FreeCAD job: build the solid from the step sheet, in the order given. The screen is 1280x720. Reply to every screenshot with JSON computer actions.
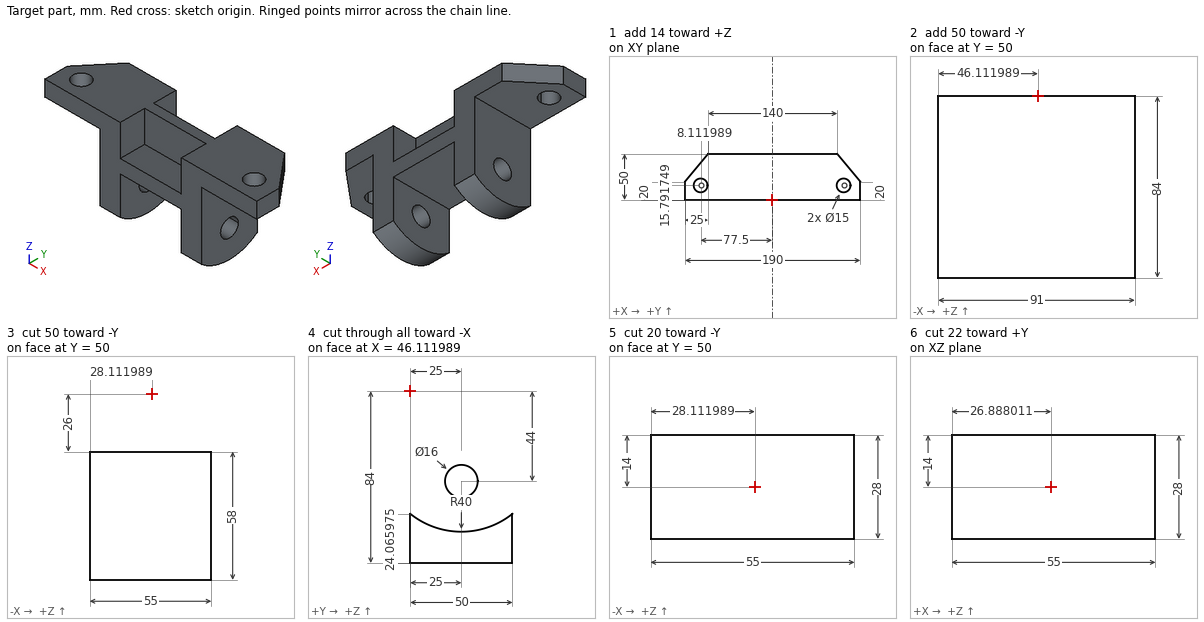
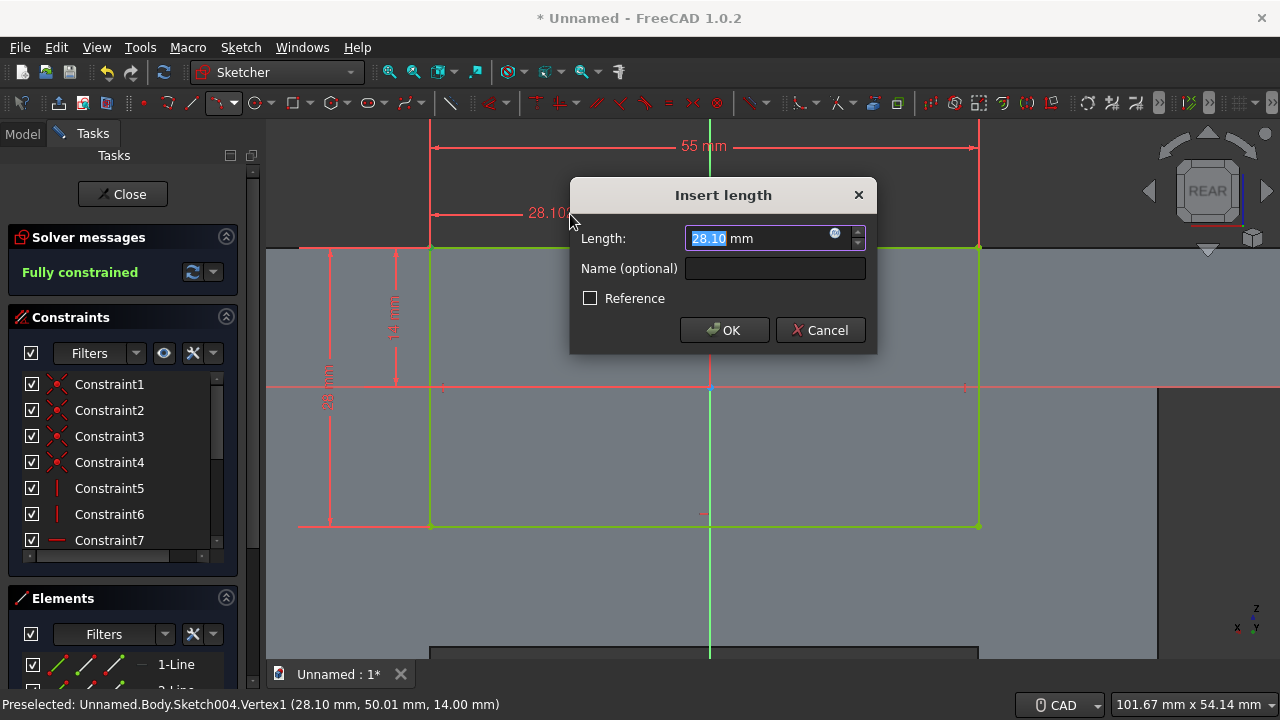
{"action": "type", "text": "28.111989"}
{"action": "key", "text": "Return"}
{"action": "key", "text": "Escape"}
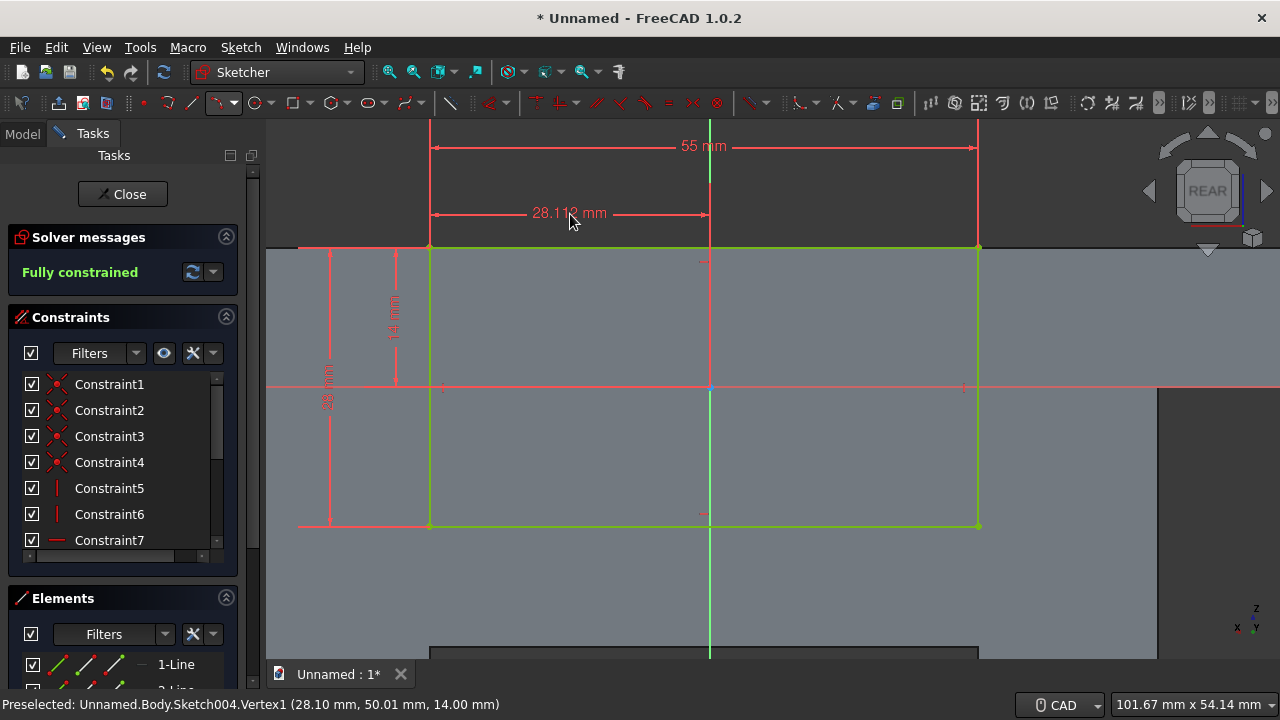
{"action": "left_click", "coordinate": [123, 194]}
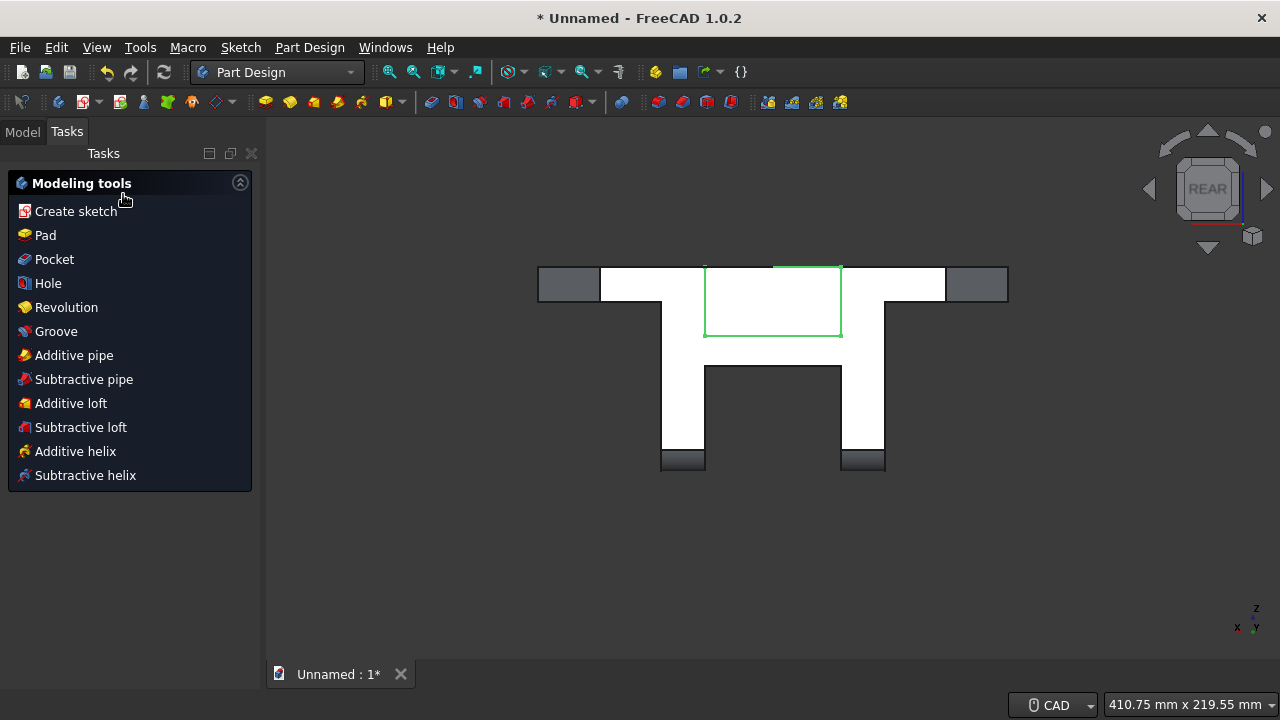
{"action": "left_click", "coordinate": [432, 102]}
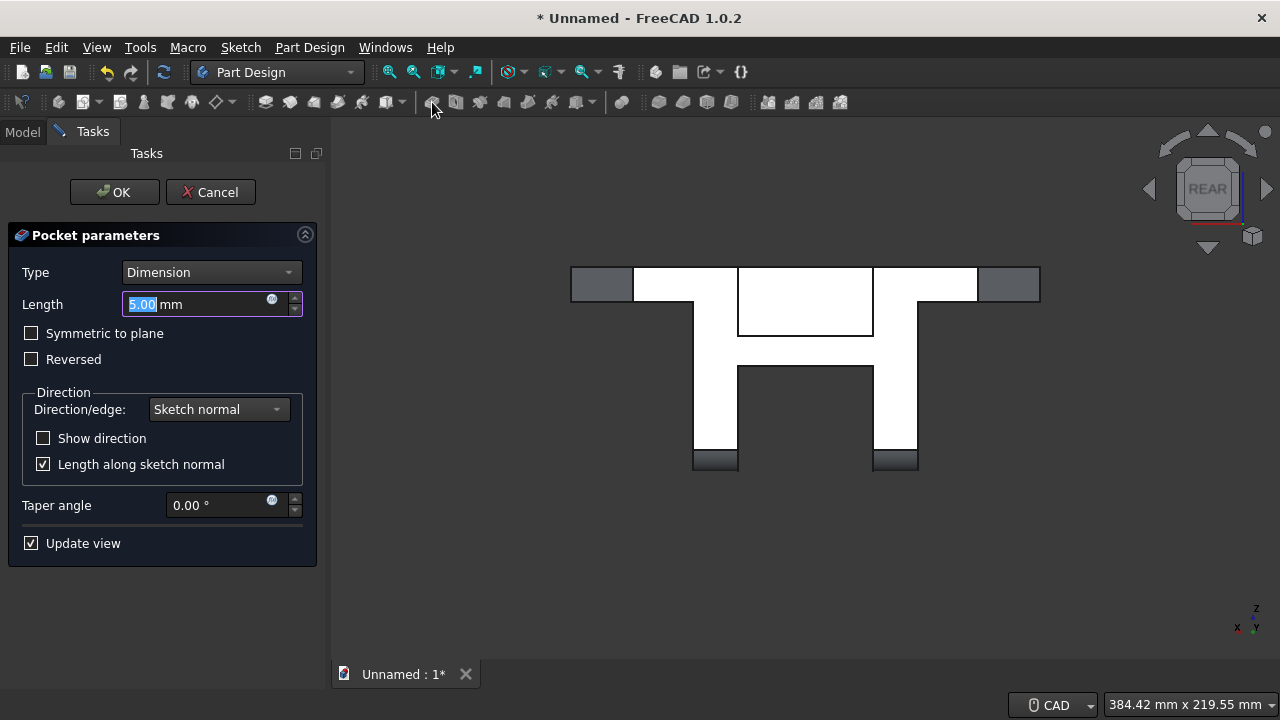
{"action": "type", "text": "20"}
{"action": "key", "text": "Tab"}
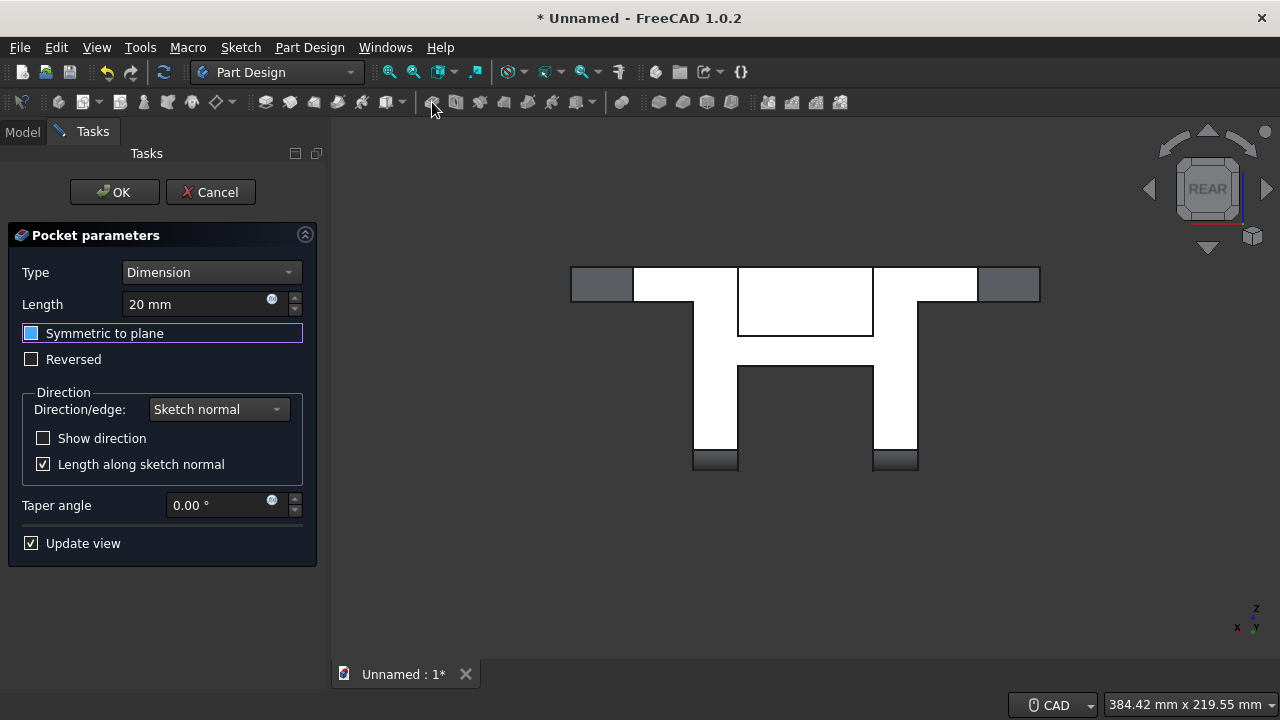
{"action": "left_click", "coordinate": [115, 192]}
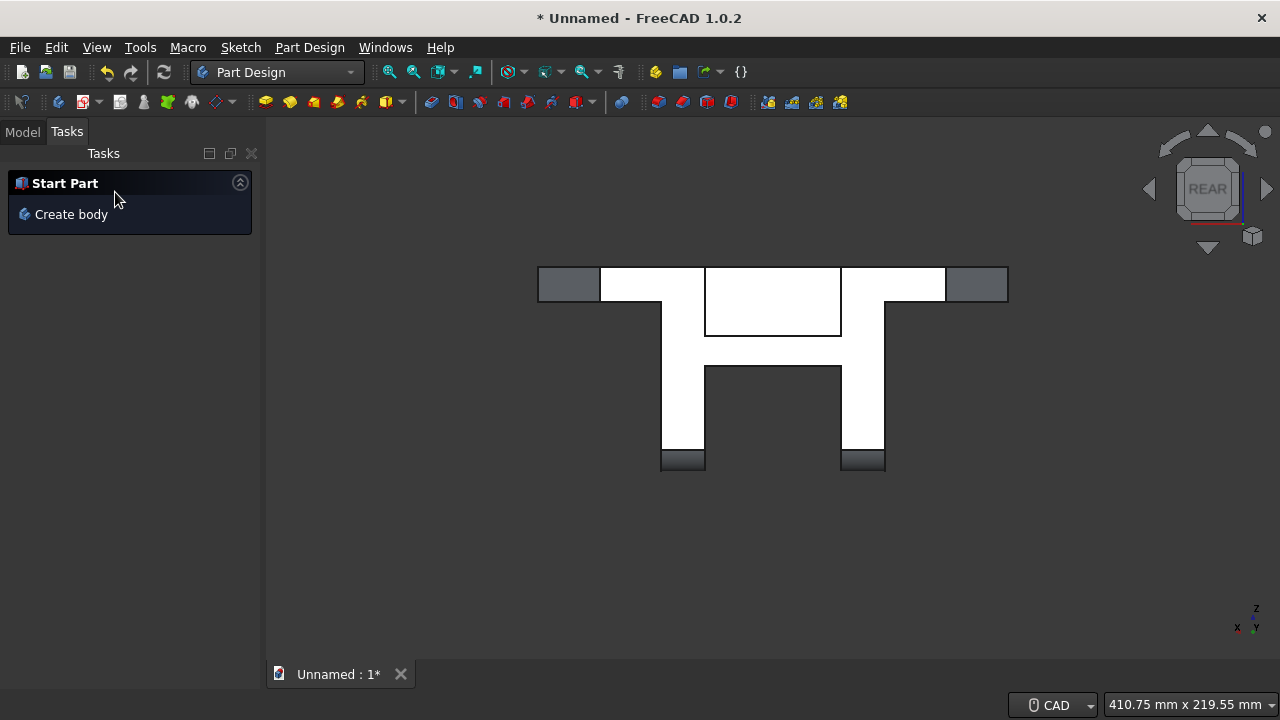
{"action": "left_click", "coordinate": [84, 102]}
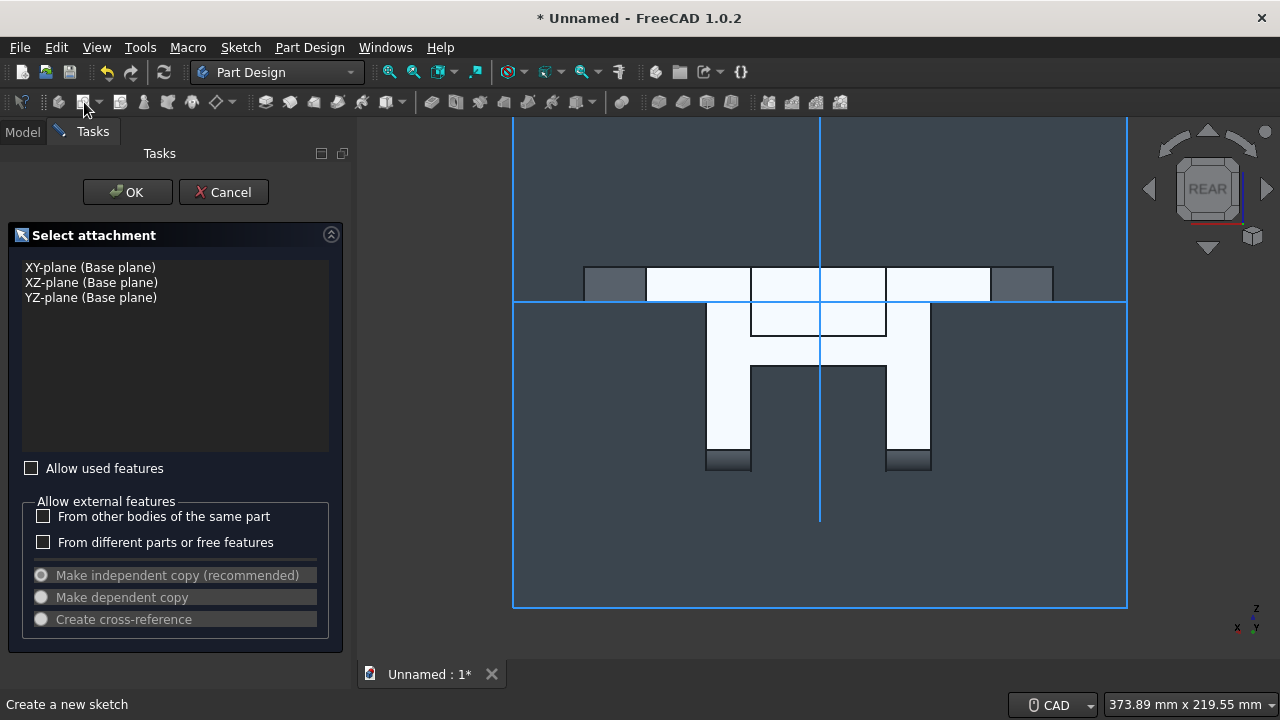
{"action": "left_click", "coordinate": [82, 282]}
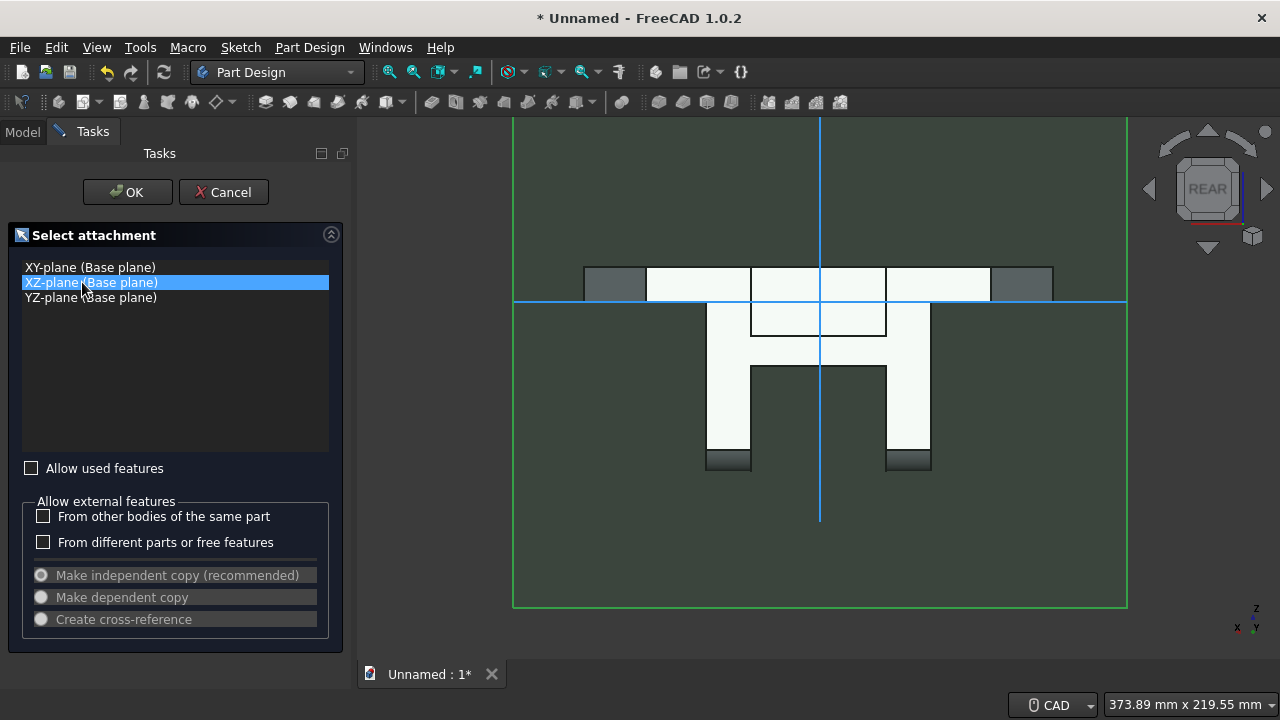
{"action": "left_click", "coordinate": [128, 192]}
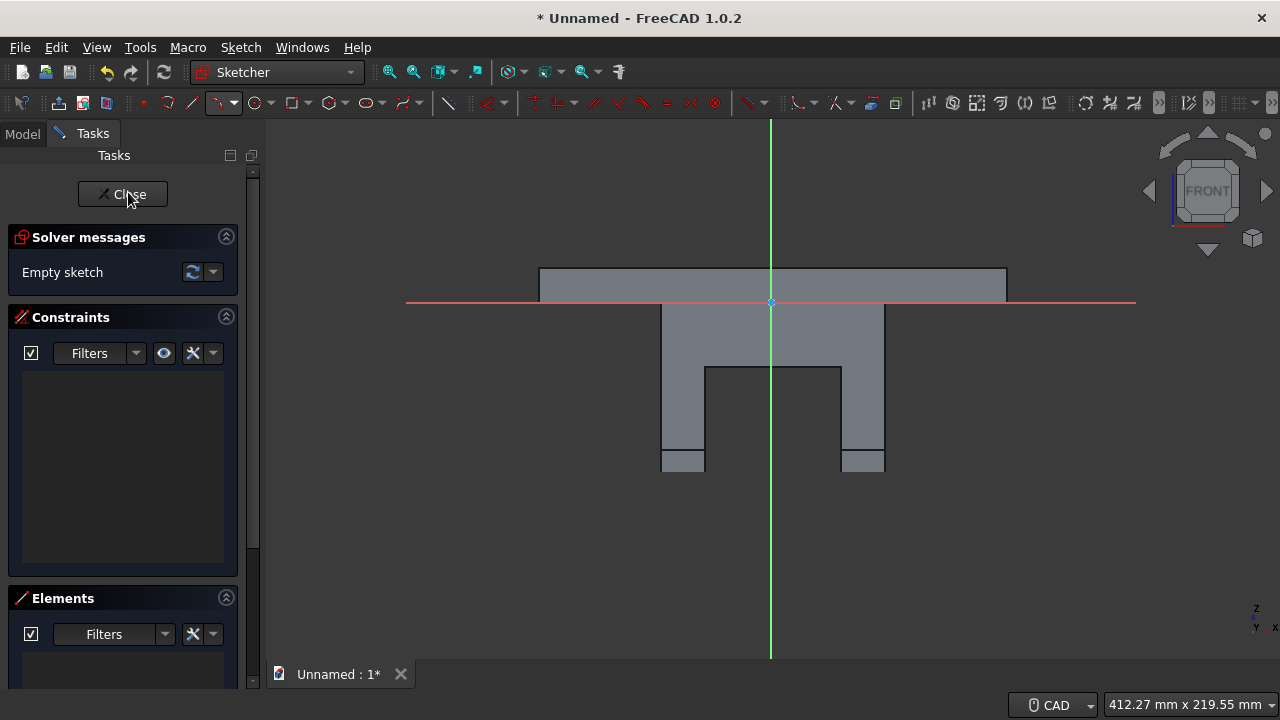
{"action": "scroll", "coordinate": [795, 275], "scroll_direction": "up", "scroll_amount": 7}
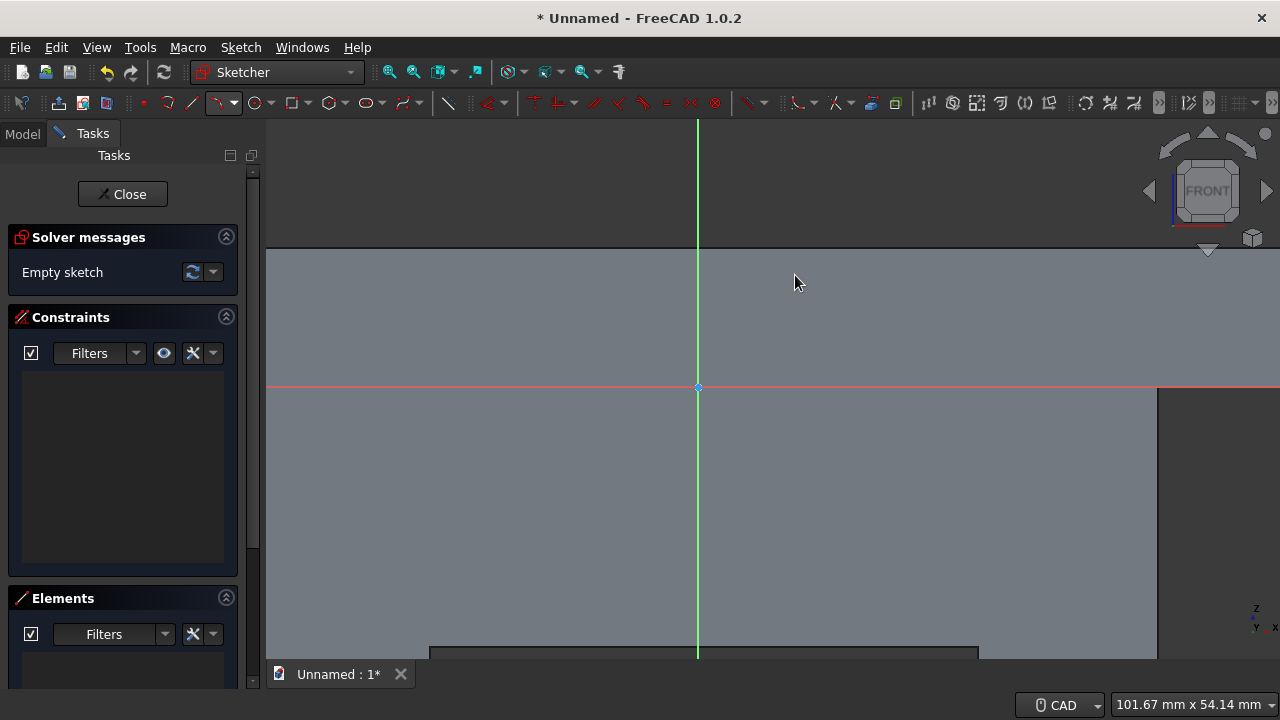
{"action": "left_click", "coordinate": [292, 104]}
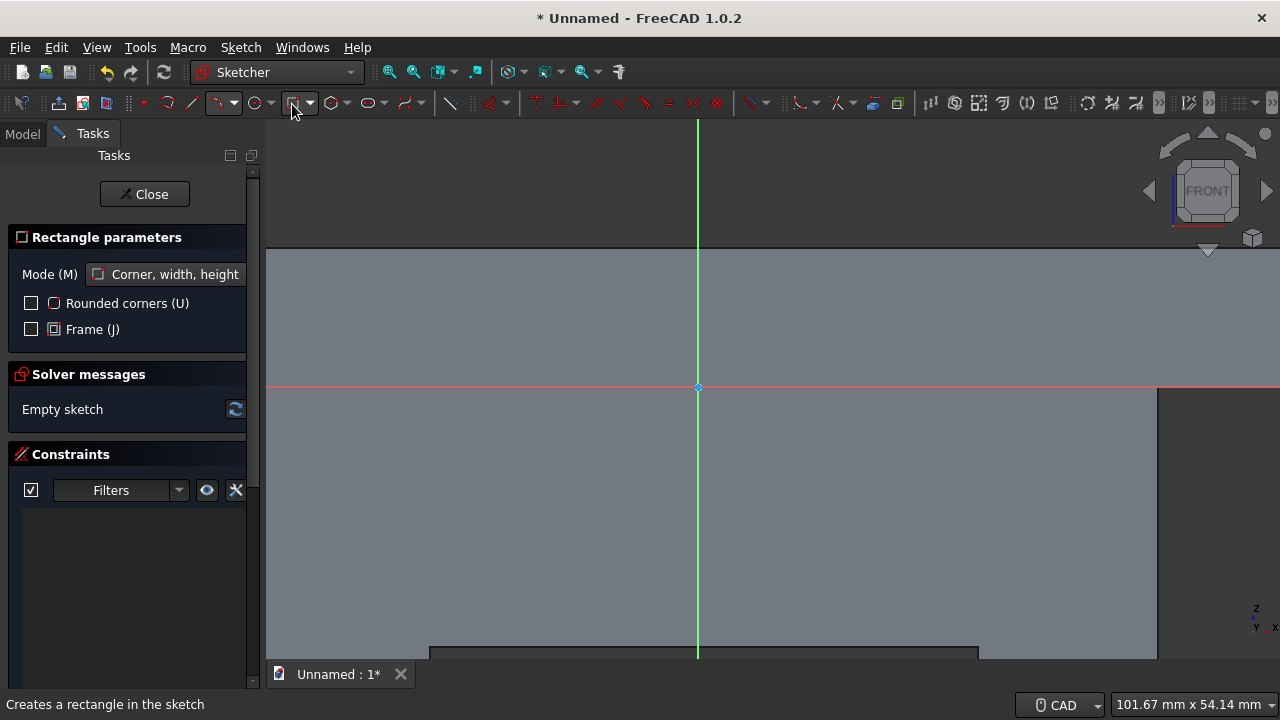
{"action": "left_click", "coordinate": [430, 248]}
{"action": "mouse_move", "coordinate": [978, 527]}